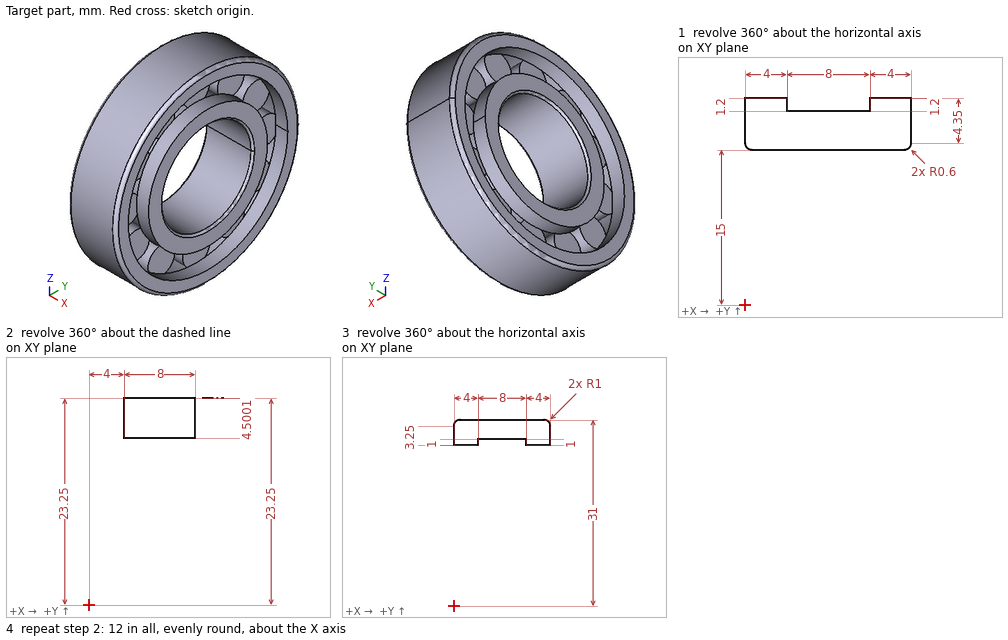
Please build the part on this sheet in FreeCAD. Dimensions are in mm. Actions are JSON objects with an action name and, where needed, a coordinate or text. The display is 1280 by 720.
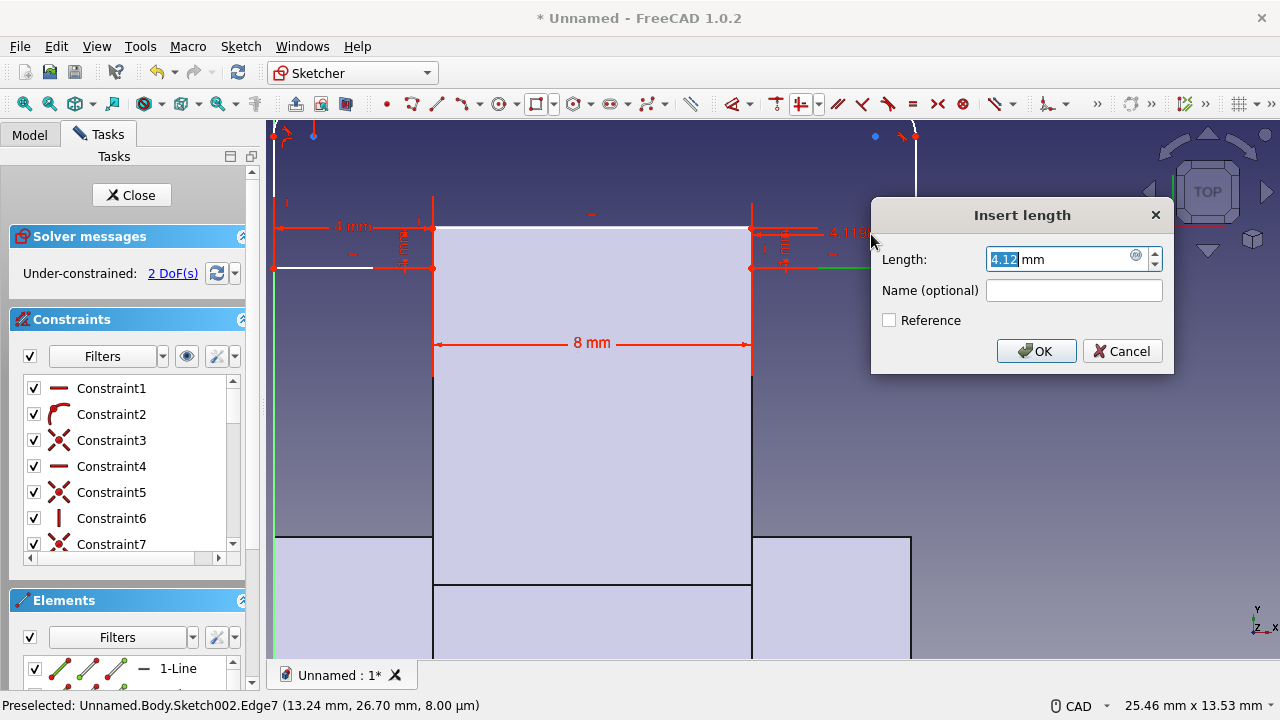
{"action": "type", "text": "4"}
{"action": "key", "text": "Return"}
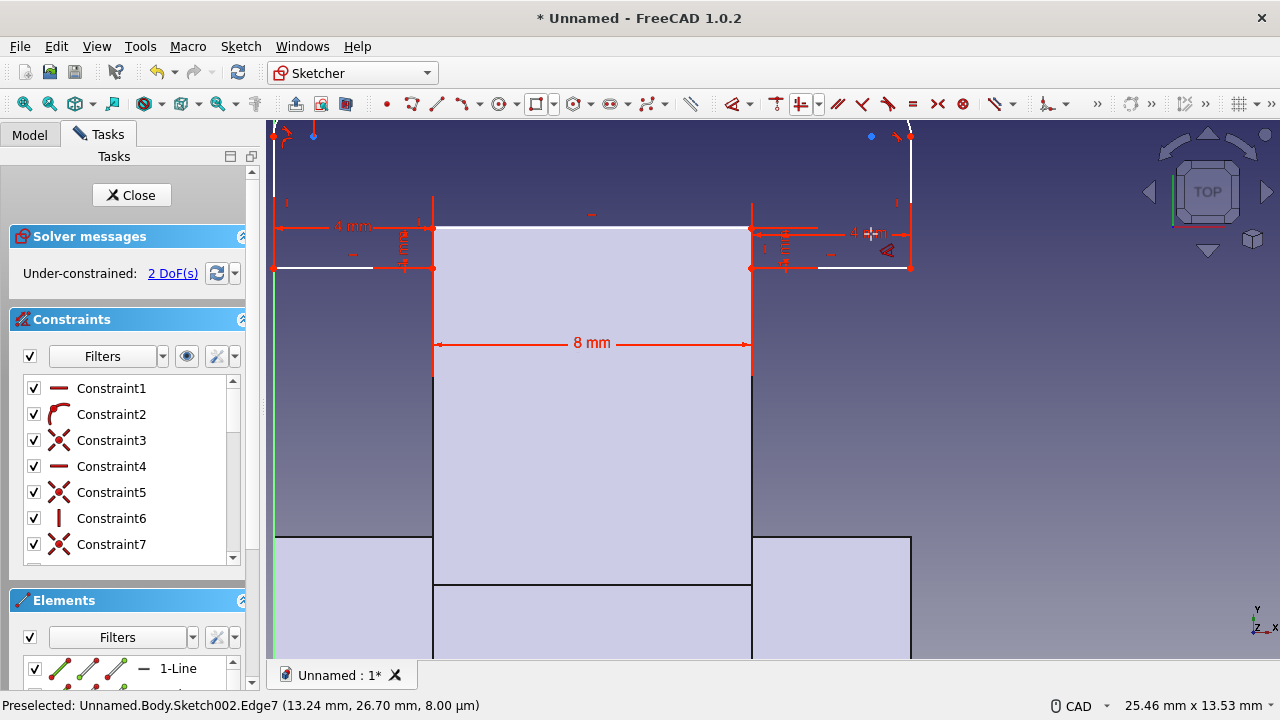
{"action": "scroll", "coordinate": [753, 249], "scroll_direction": "down", "scroll_amount": 6}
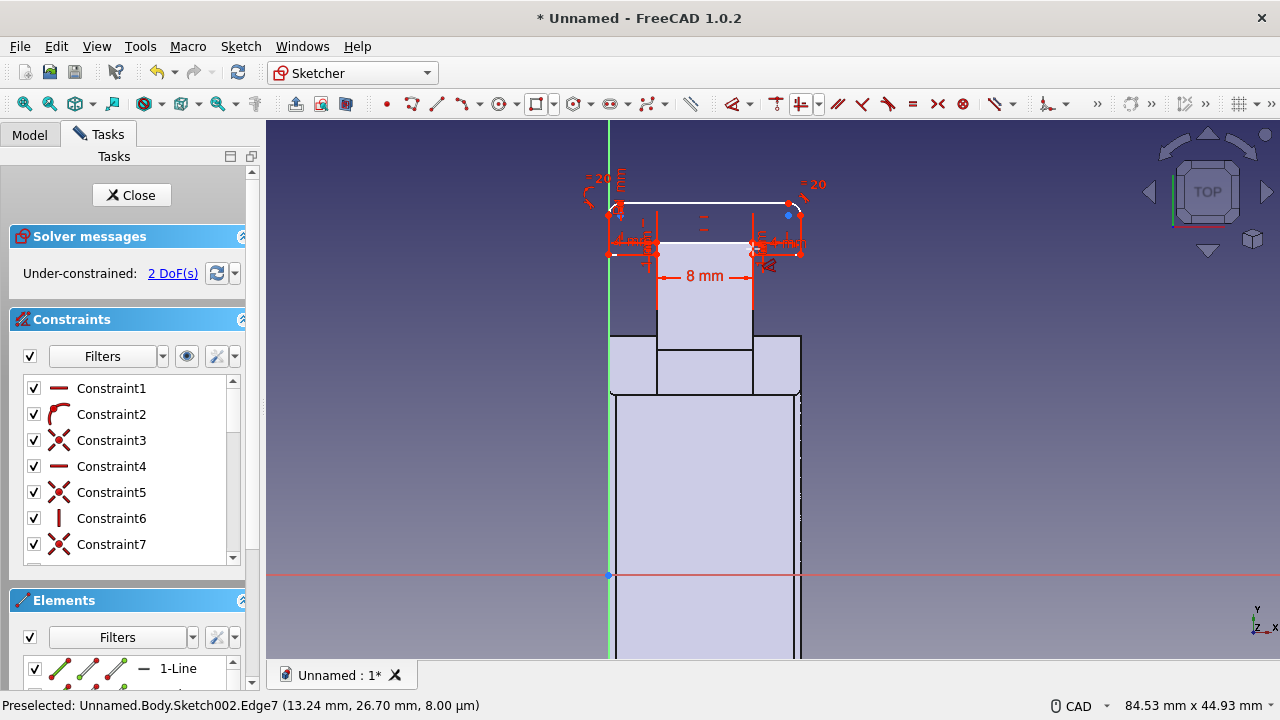
{"action": "left_click", "coordinate": [789, 203]}
{"action": "left_click", "coordinate": [575, 389]}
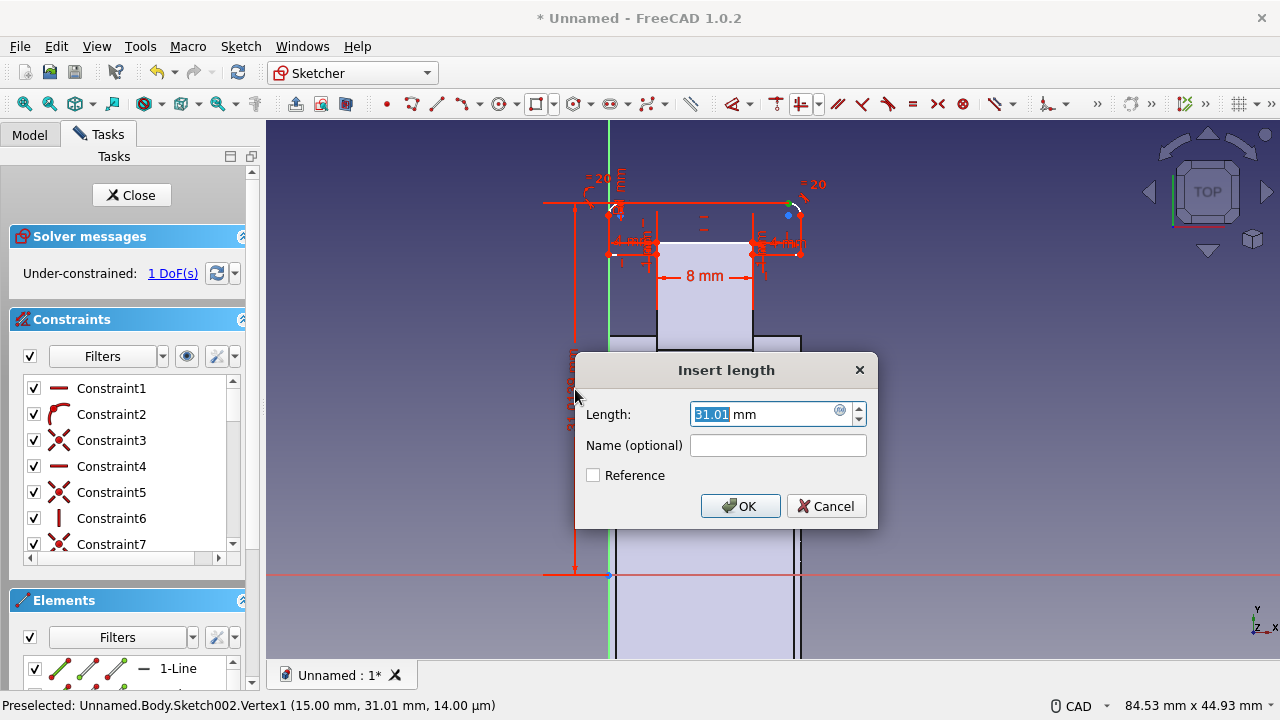
{"action": "type", "text": "31"}
{"action": "key", "text": "Return"}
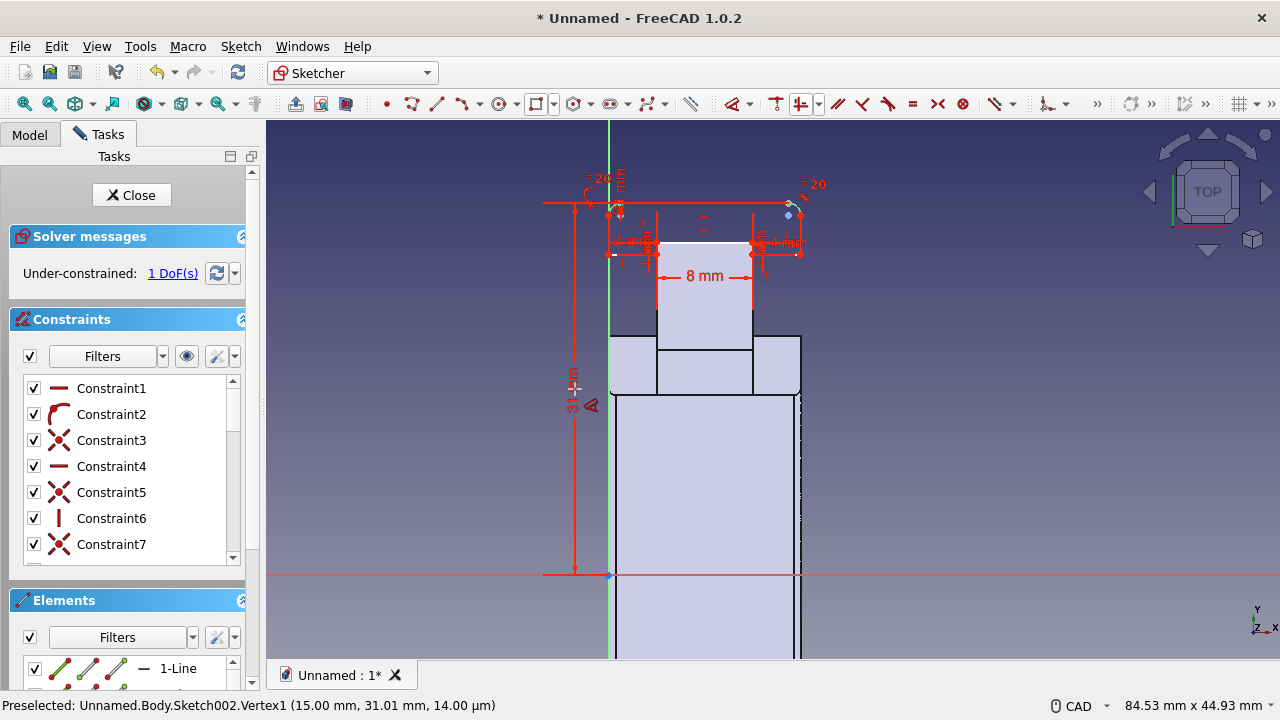
{"action": "left_click", "coordinate": [609, 227]}
{"action": "left_click", "coordinate": [575, 221]}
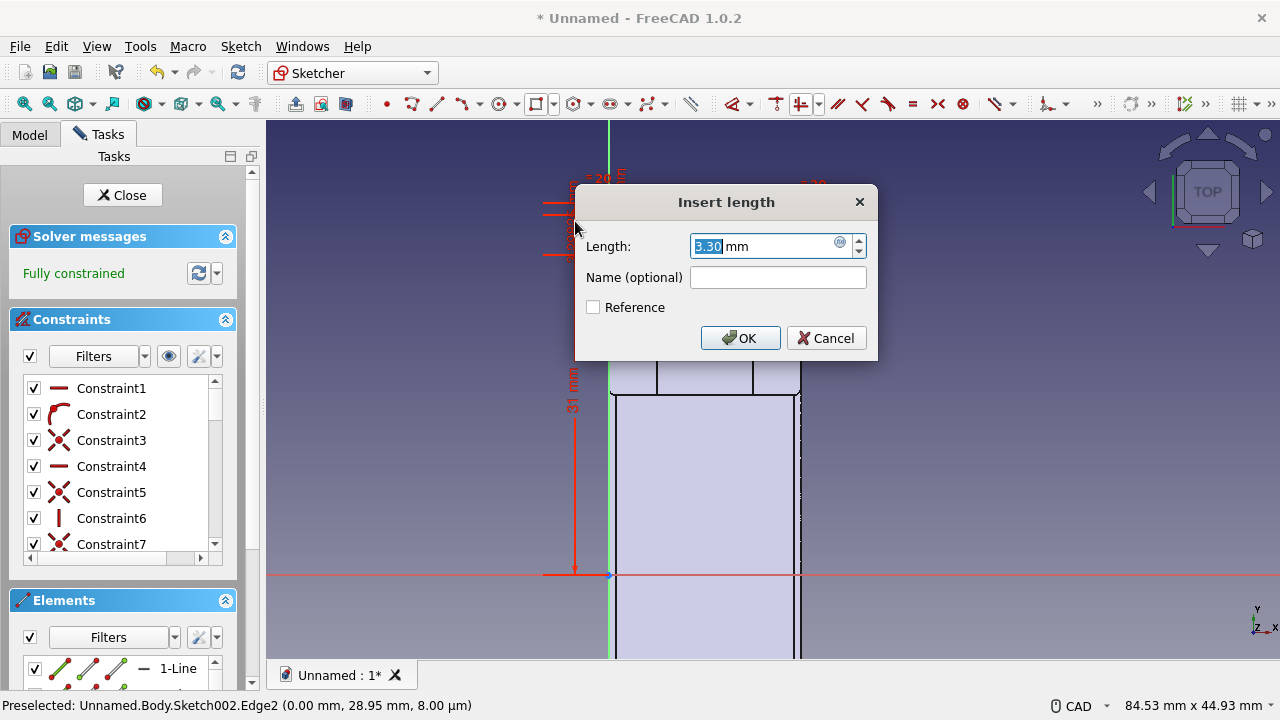
{"action": "type", "text": "3.25"}
{"action": "key", "text": "Return"}
{"action": "key", "text": "Escape"}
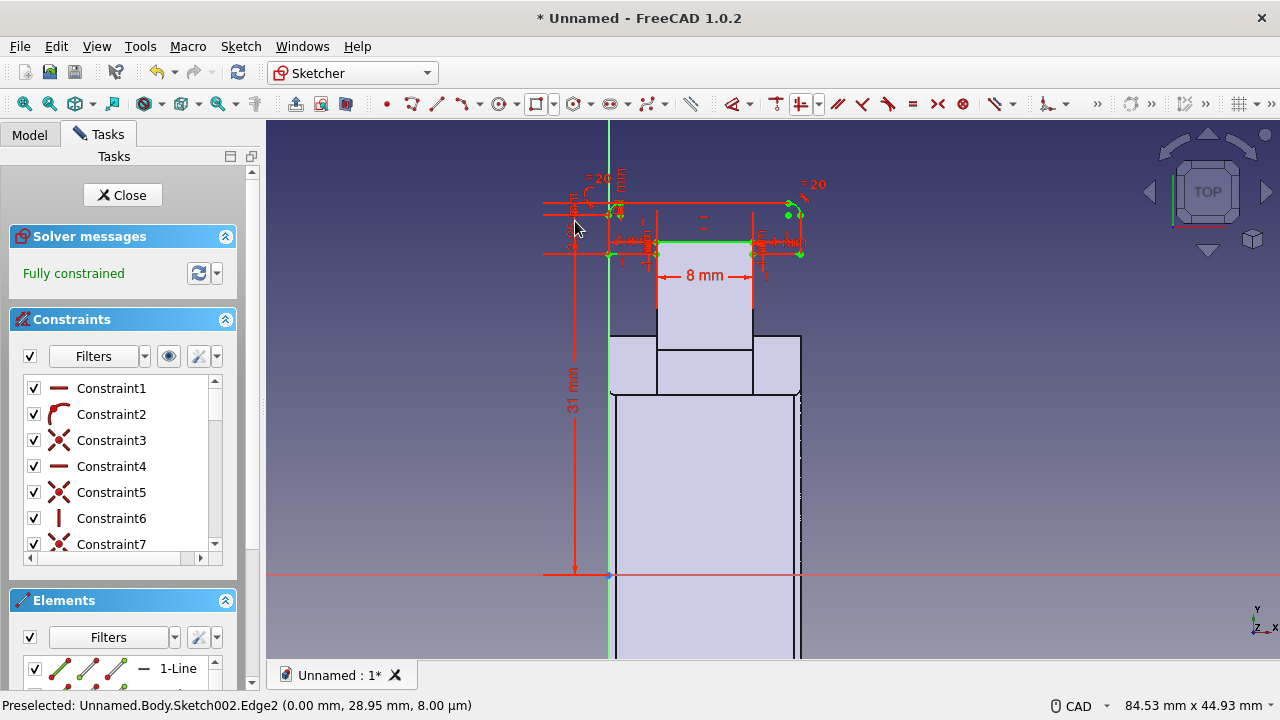
{"action": "left_click", "coordinate": [123, 195]}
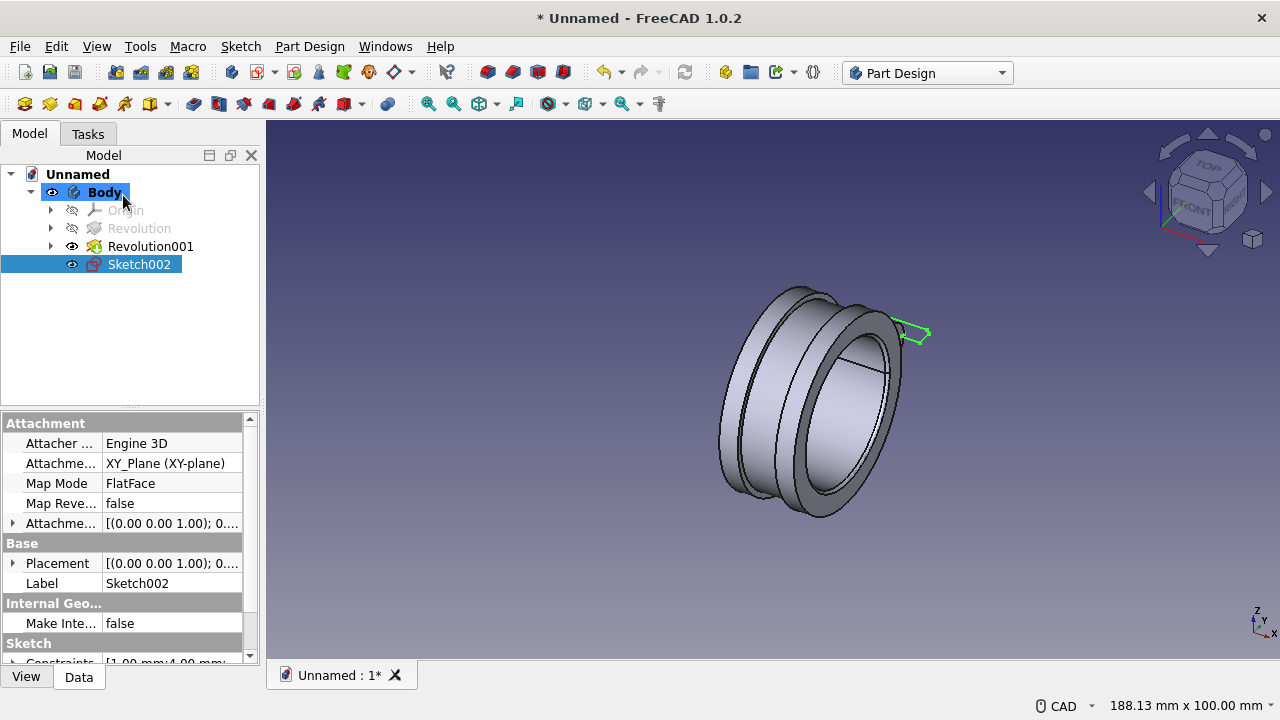
{"action": "left_click", "coordinate": [50, 104]}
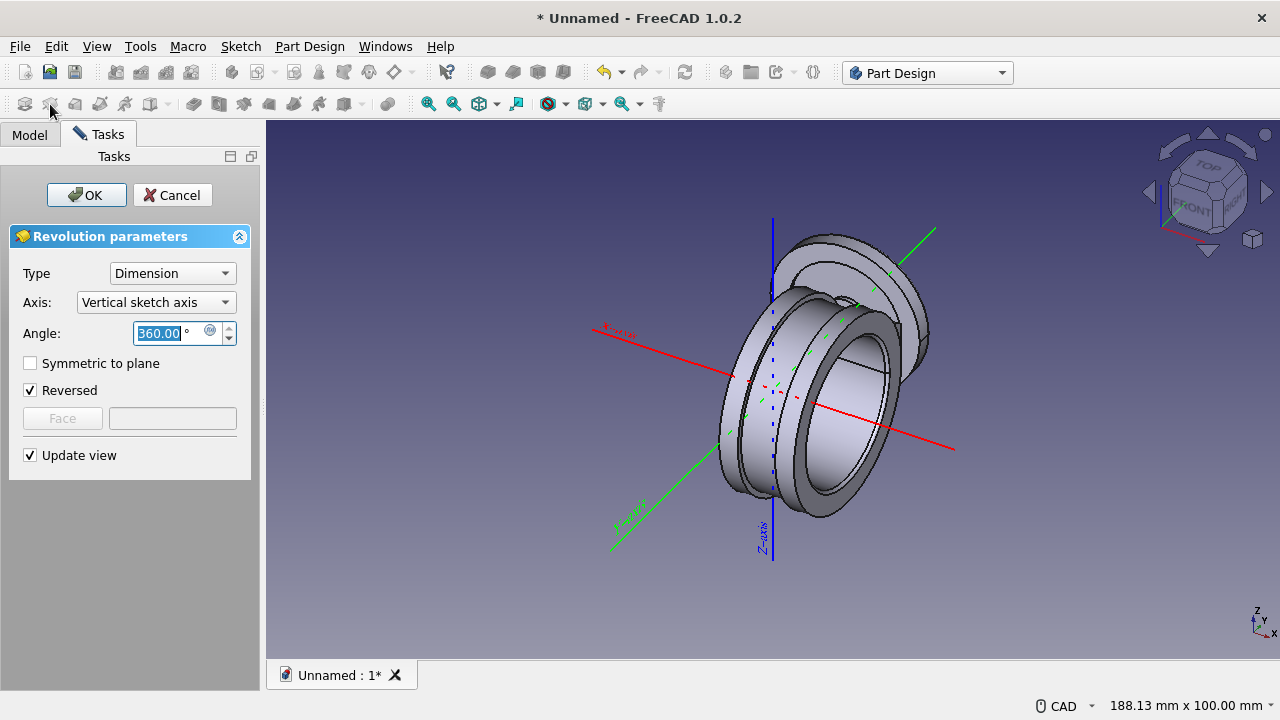
{"action": "left_click", "coordinate": [157, 302]}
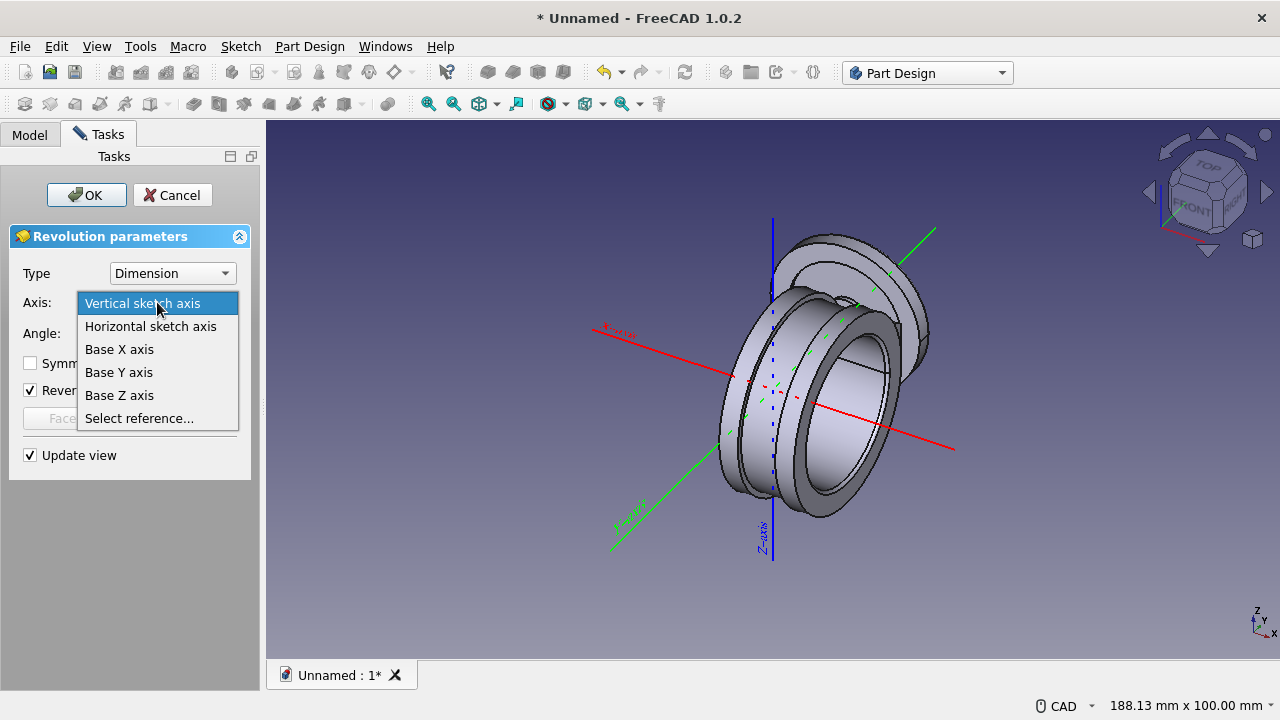
{"action": "left_click", "coordinate": [156, 326]}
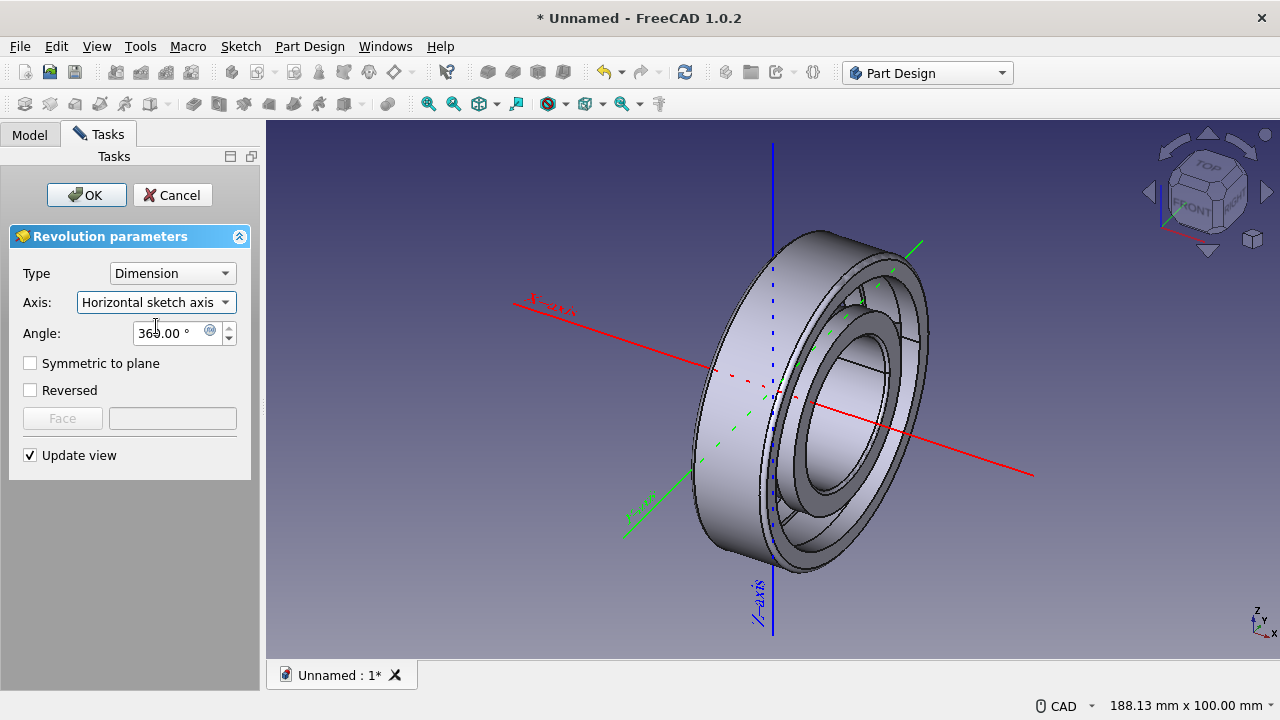
{"action": "left_click", "coordinate": [87, 195]}